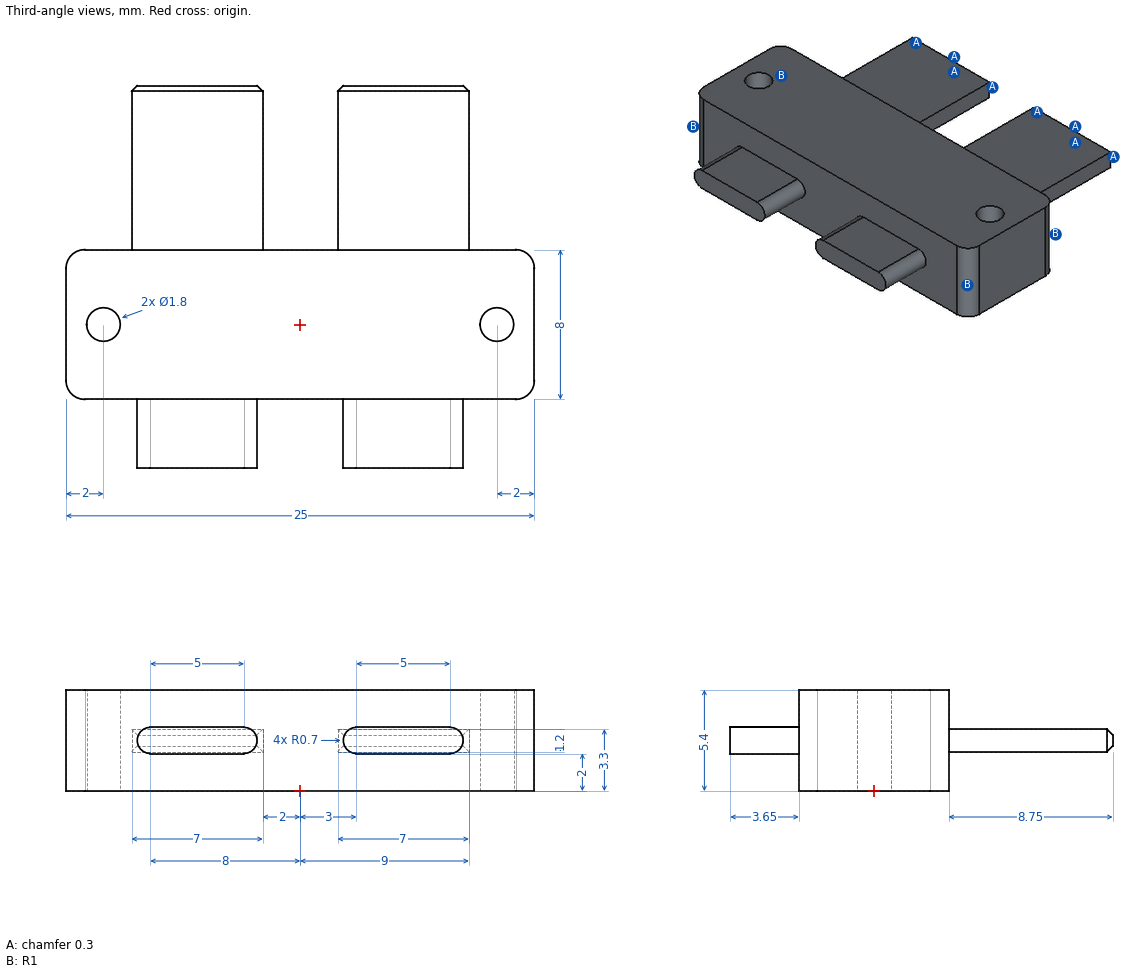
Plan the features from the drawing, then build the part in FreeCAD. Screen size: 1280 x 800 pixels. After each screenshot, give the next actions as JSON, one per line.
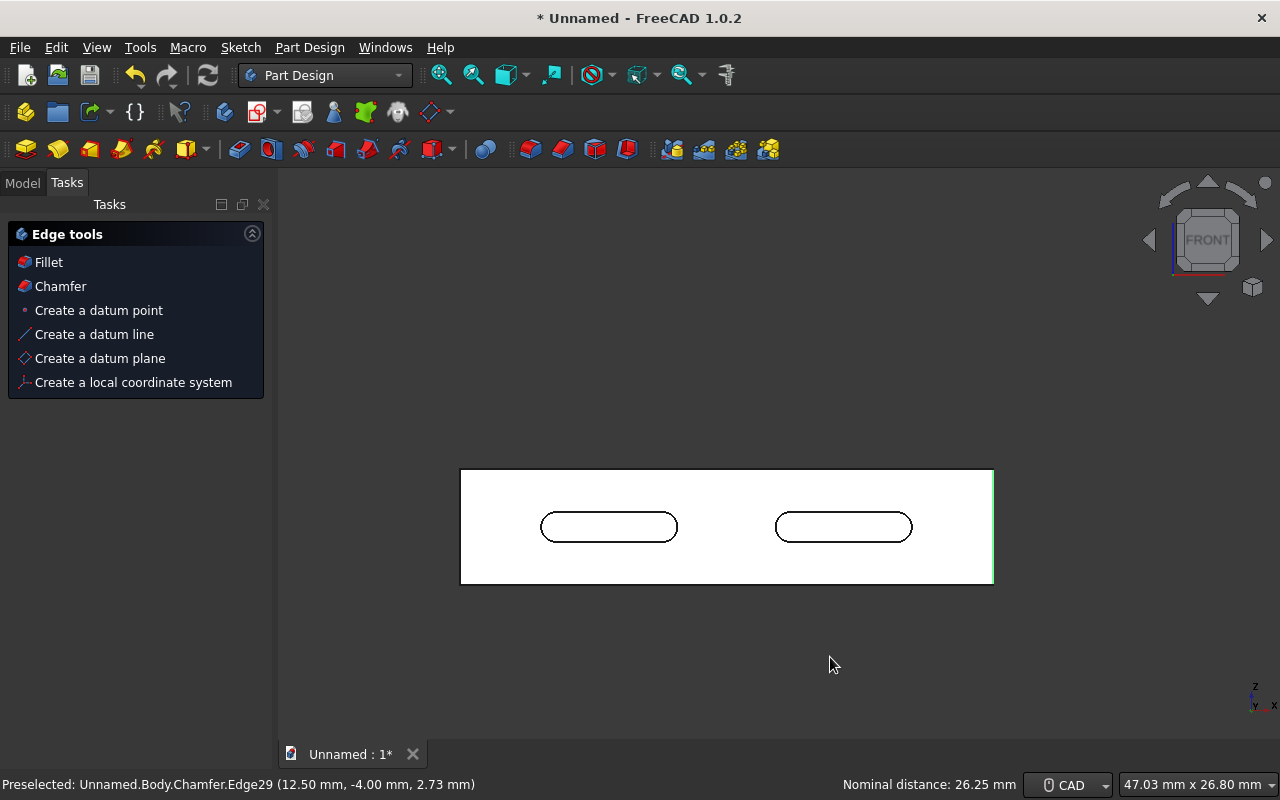
{"action": "left_click", "coordinate": [460, 526], "text": "ctrl"}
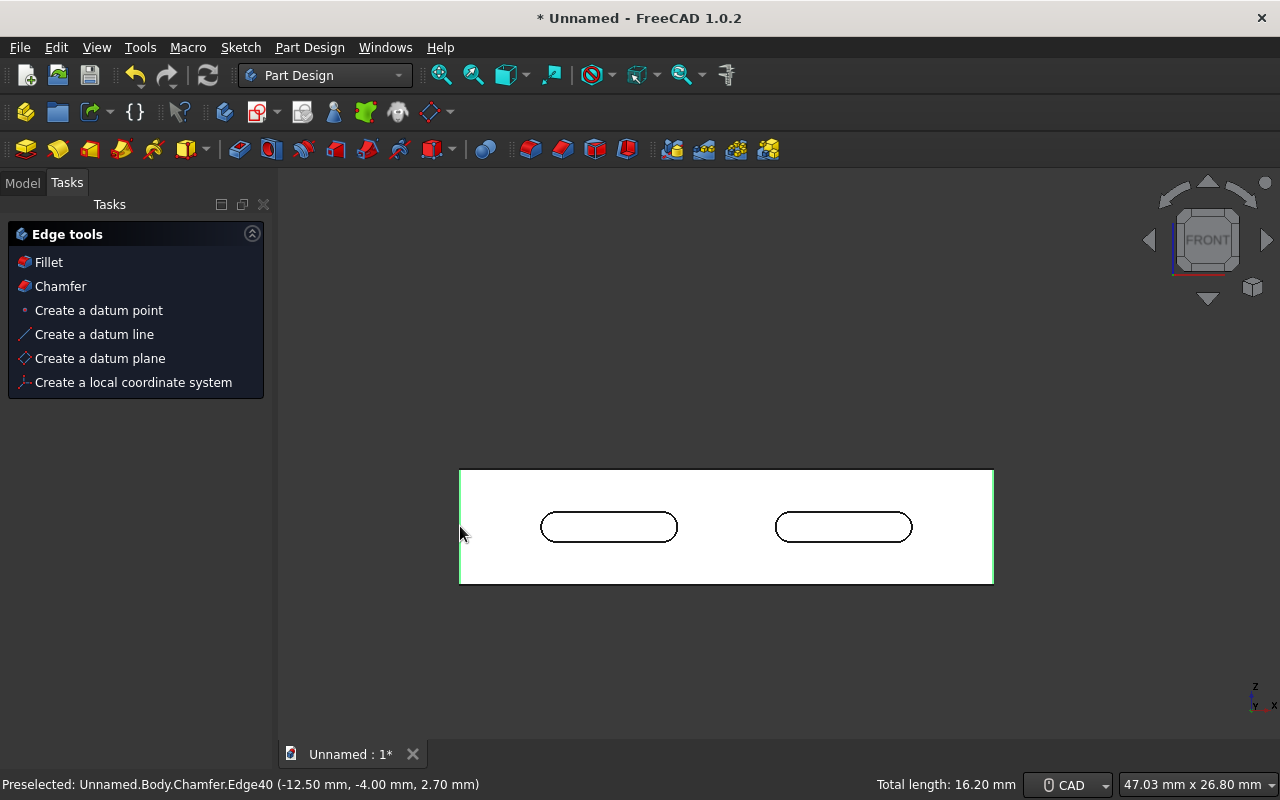
{"action": "key", "text": "3"}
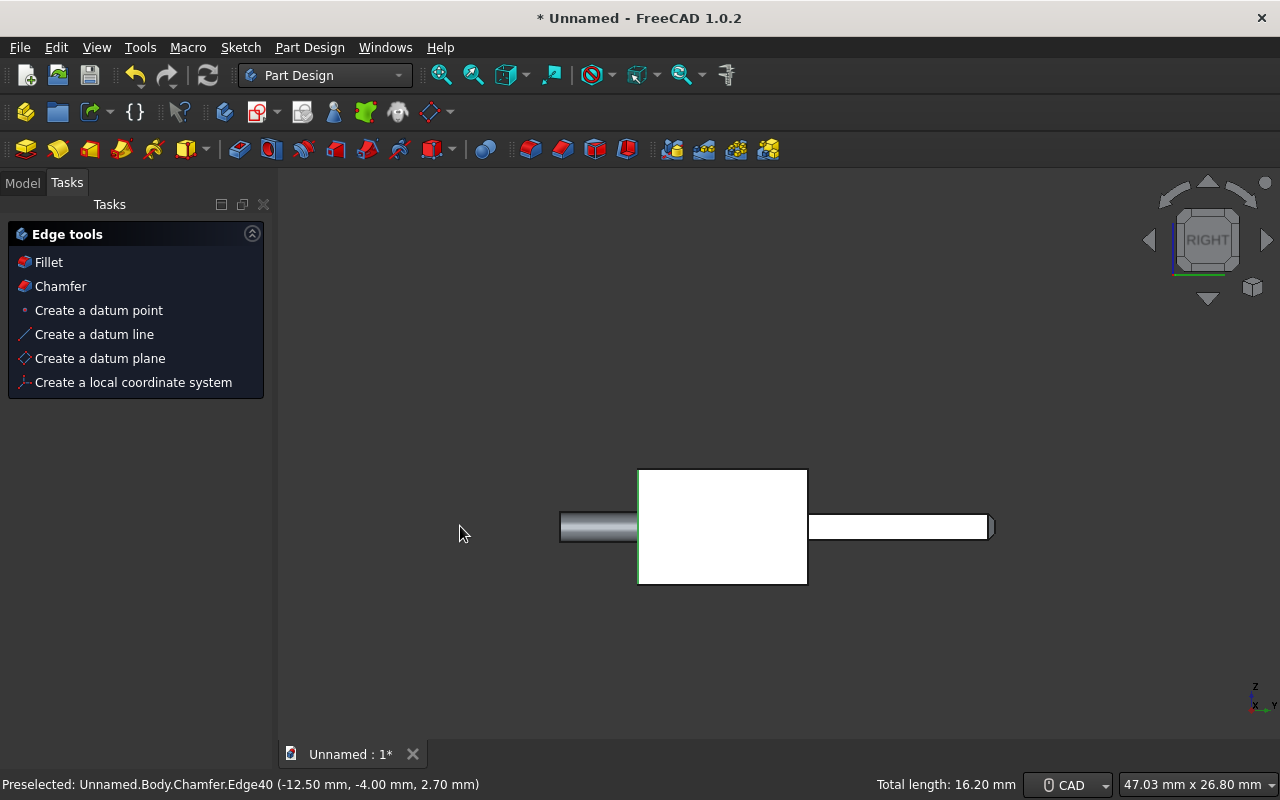
{"action": "left_click", "coordinate": [442, 76]}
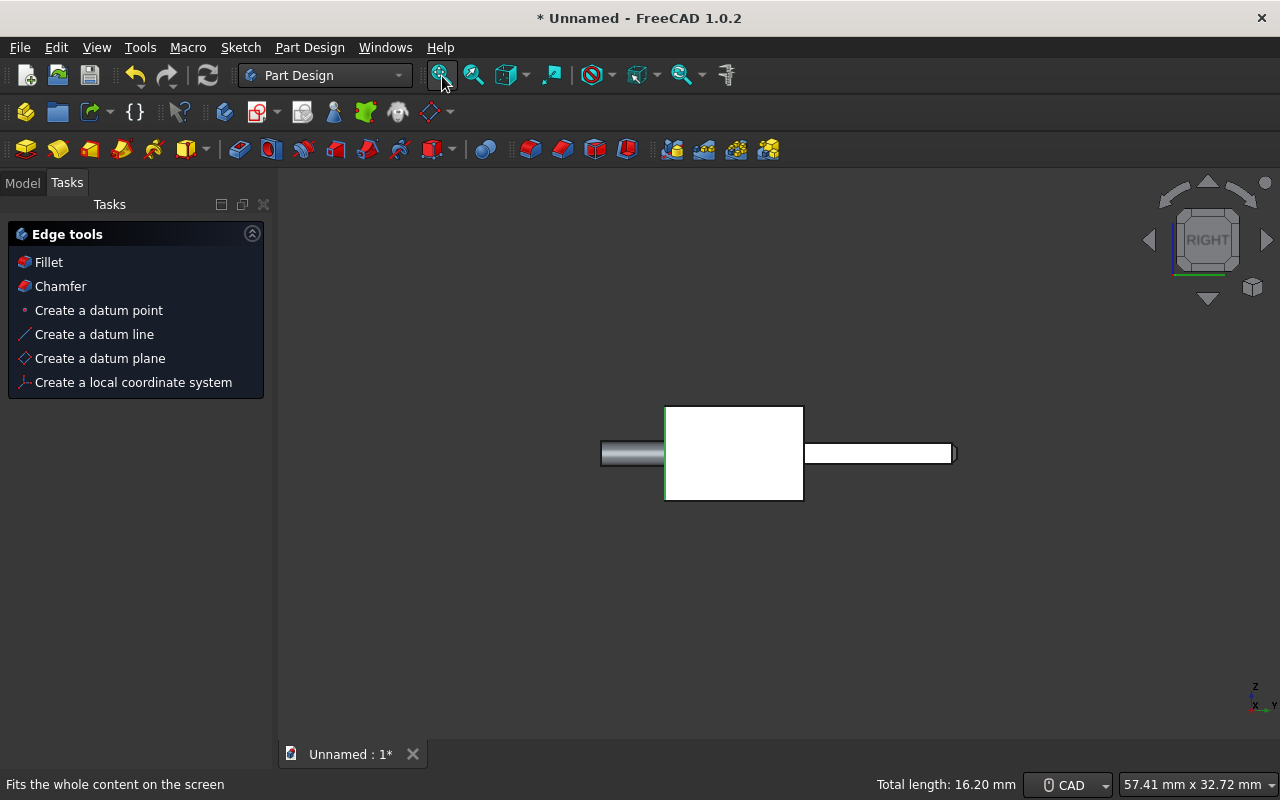
{"action": "left_click", "coordinate": [804, 452], "text": "ctrl"}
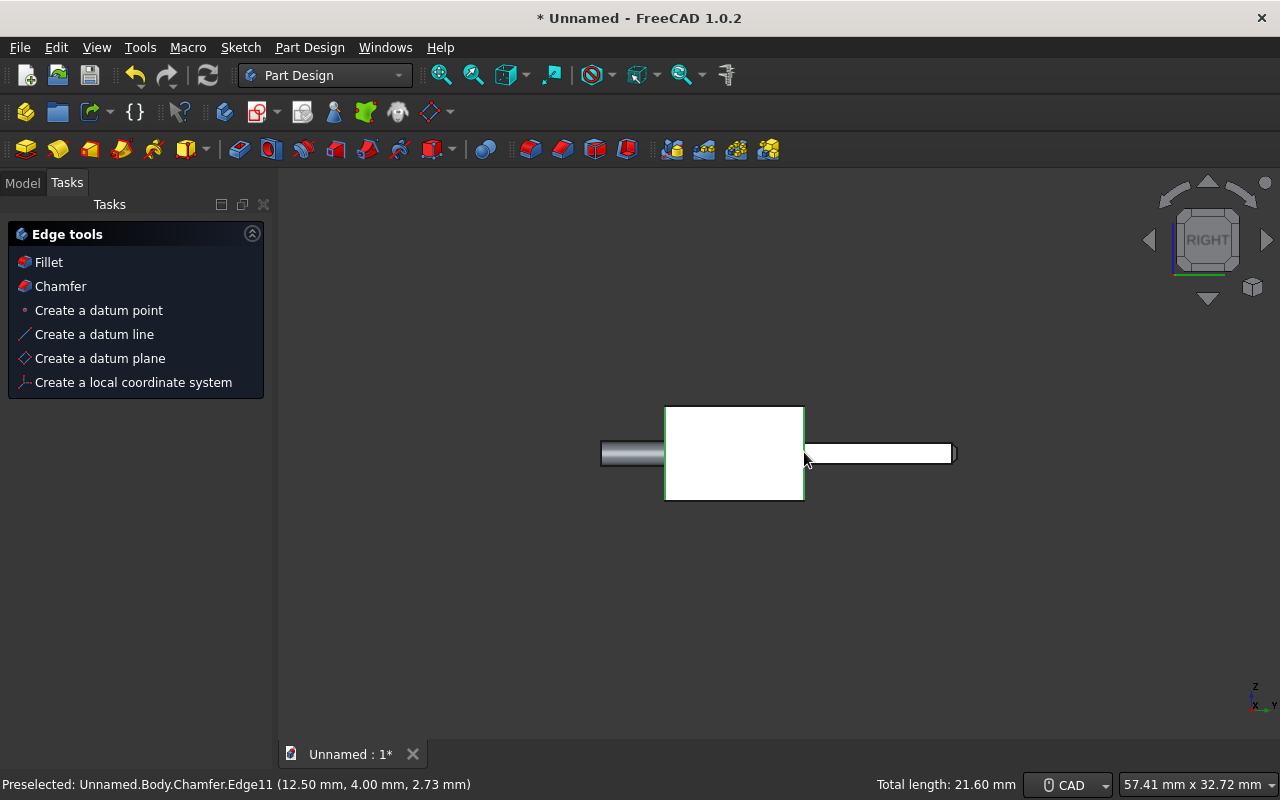
{"action": "left_click", "coordinate": [532, 150]}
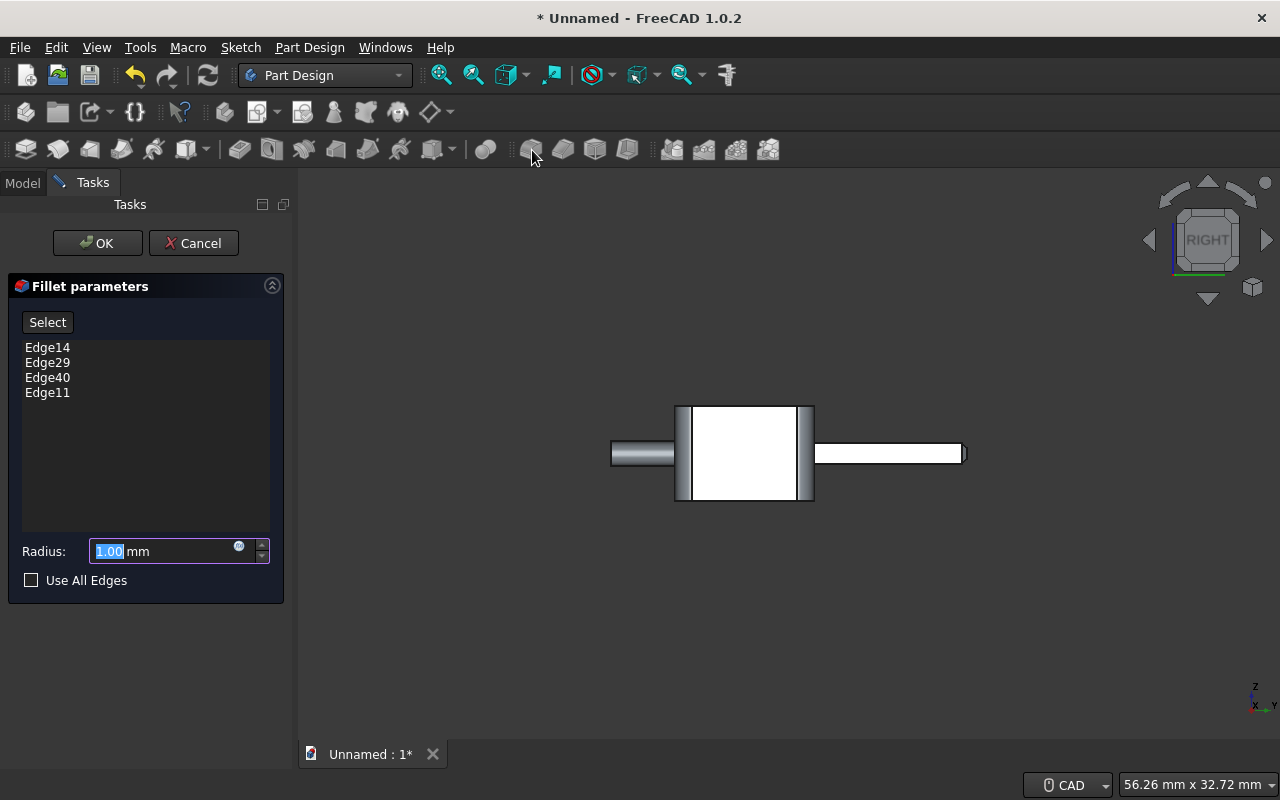
{"action": "type", "text": "1"}
{"action": "key", "text": "Tab"}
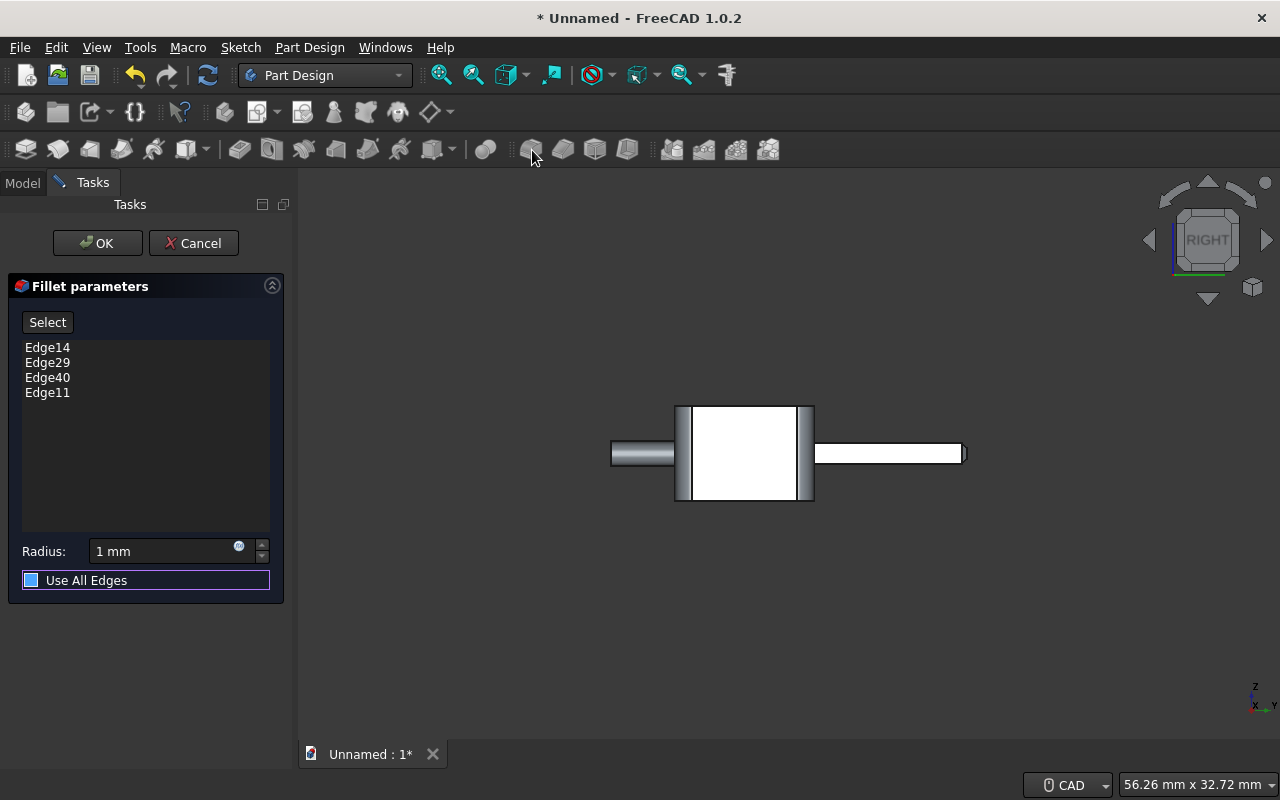
{"action": "left_click", "coordinate": [98, 243]}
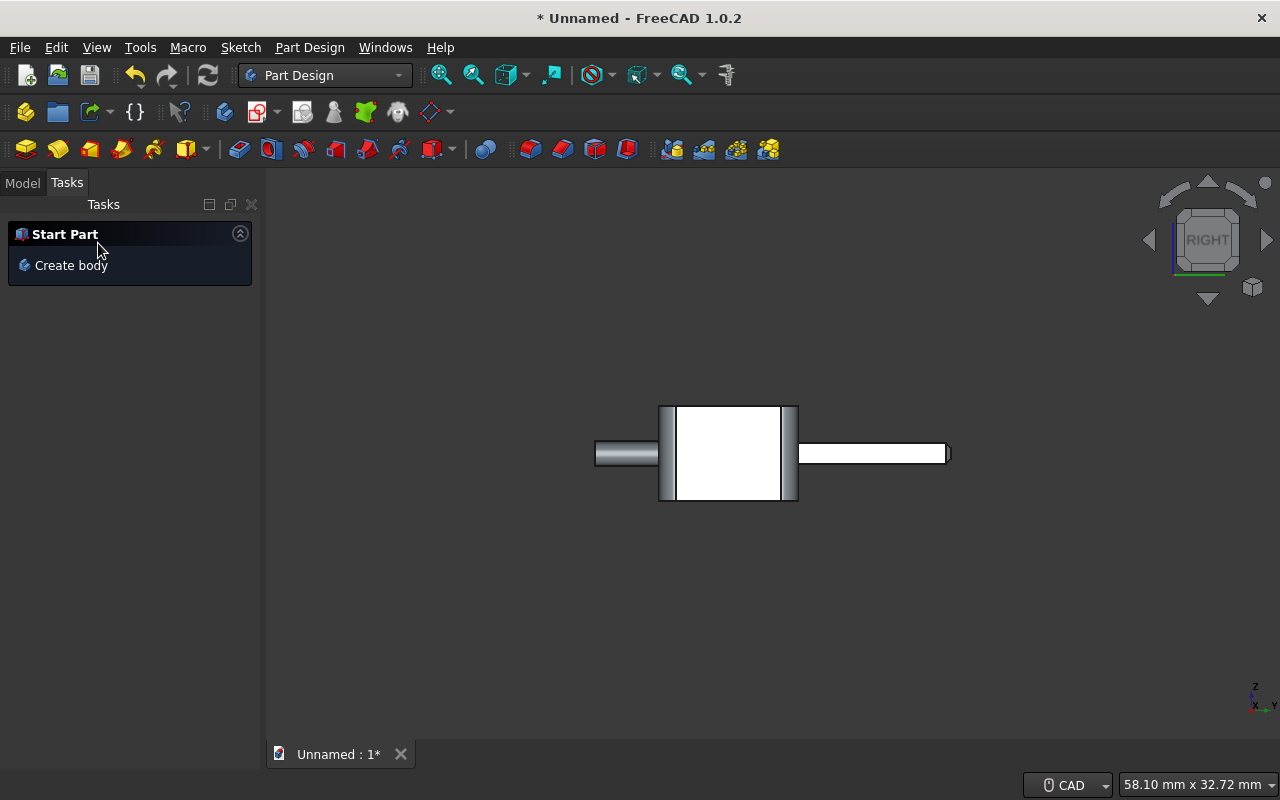
{"action": "key", "text": "0"}